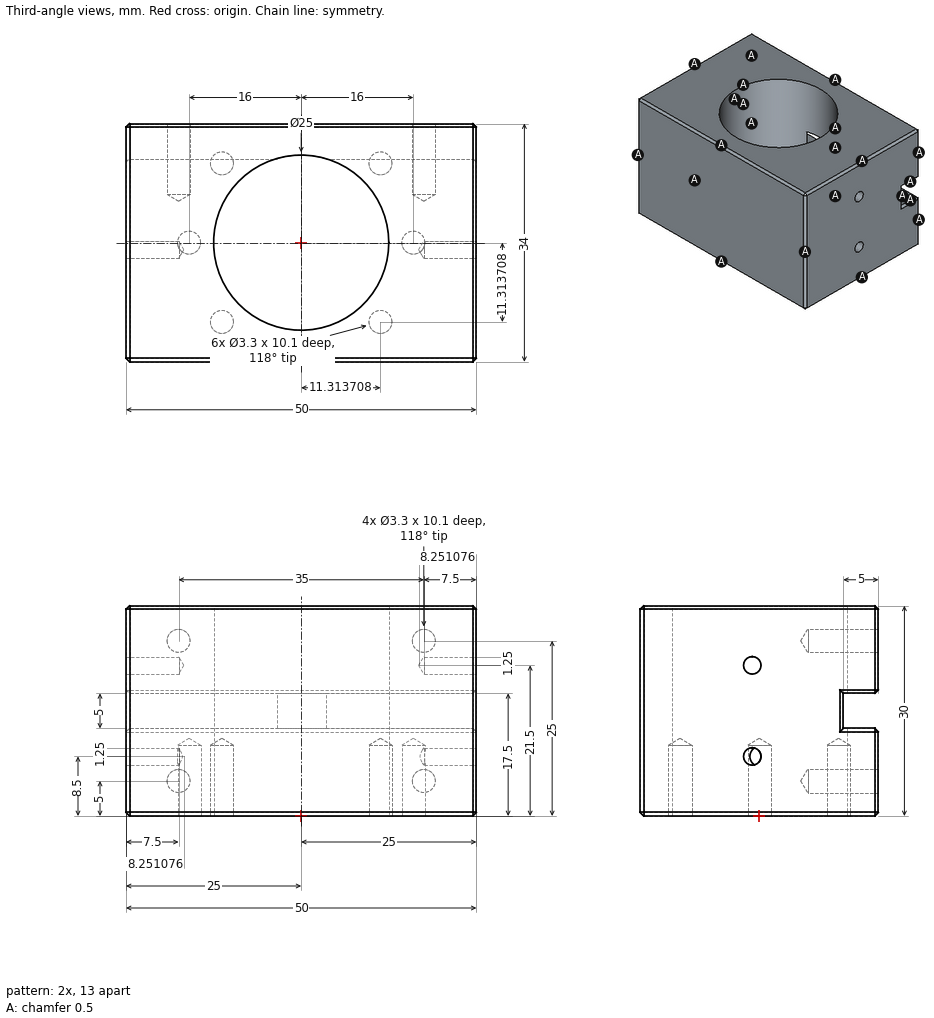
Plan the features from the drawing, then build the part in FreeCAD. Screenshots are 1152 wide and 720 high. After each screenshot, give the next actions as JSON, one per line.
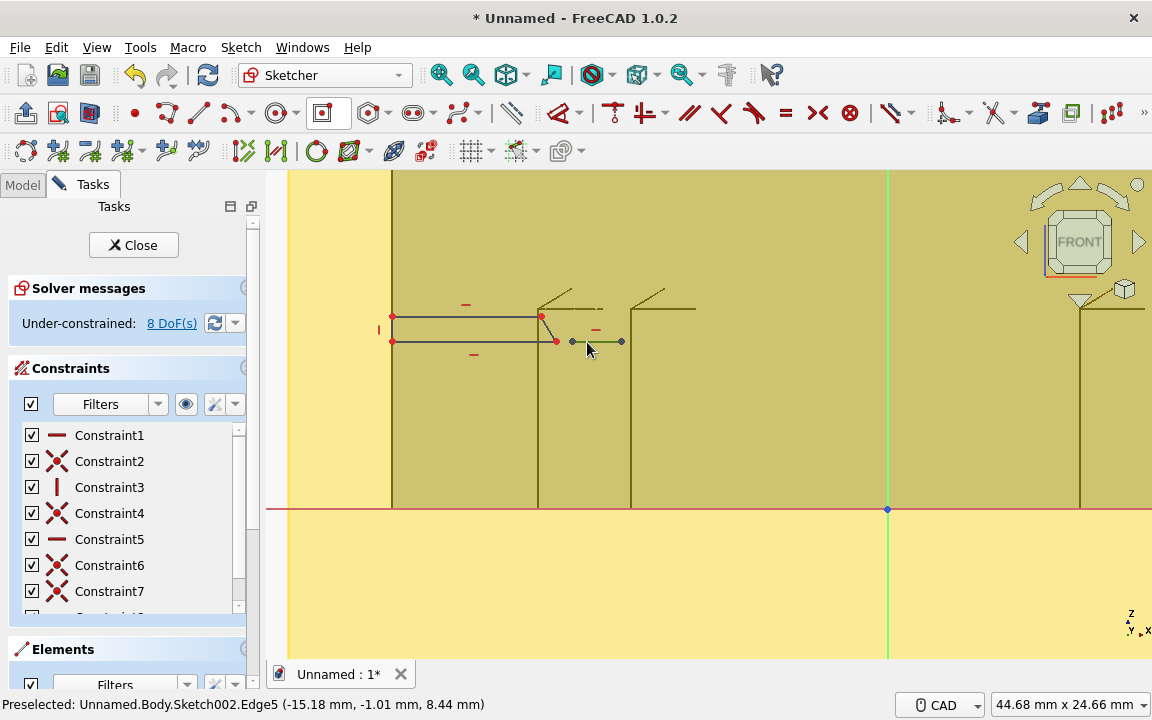
{"action": "left_click", "coordinate": [512, 114]}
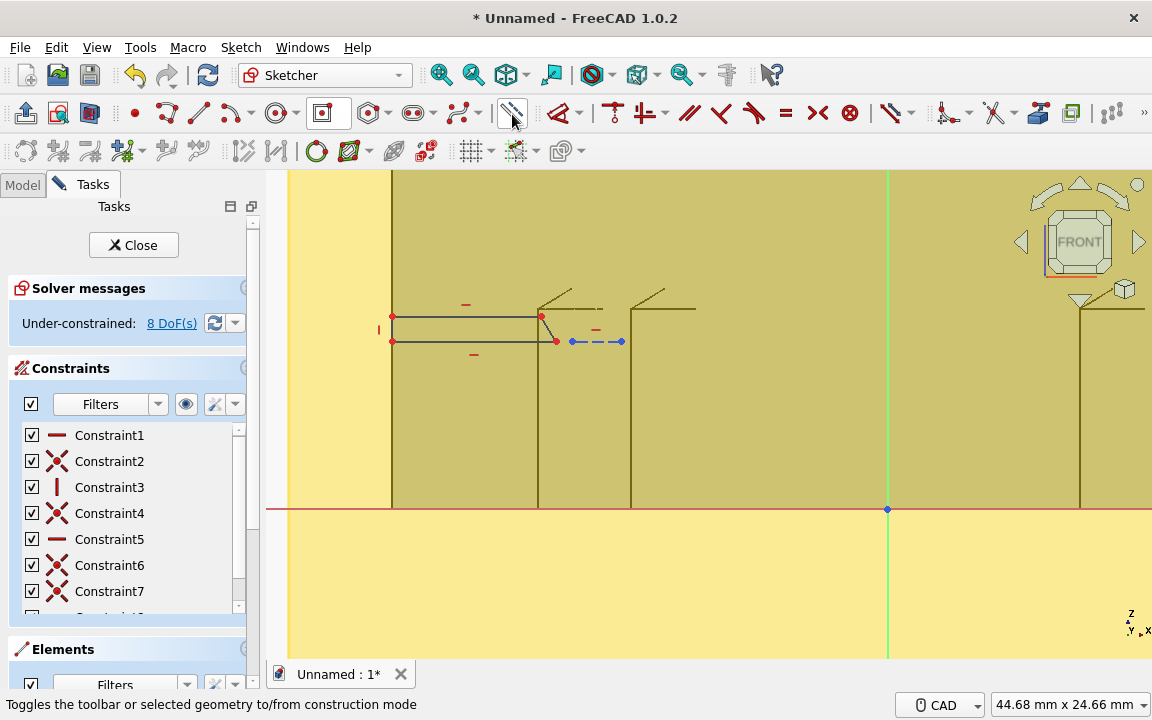
{"action": "left_click", "coordinate": [558, 114]}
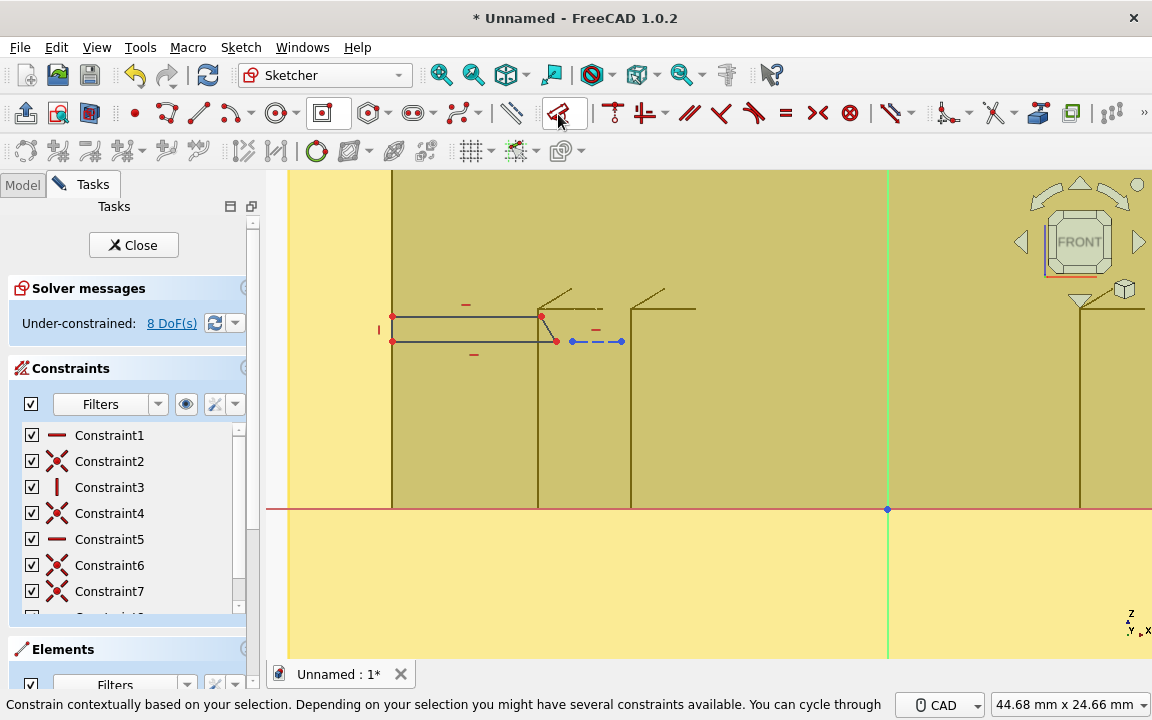
{"action": "left_click", "coordinate": [437, 317]}
{"action": "left_click", "coordinate": [466, 283]}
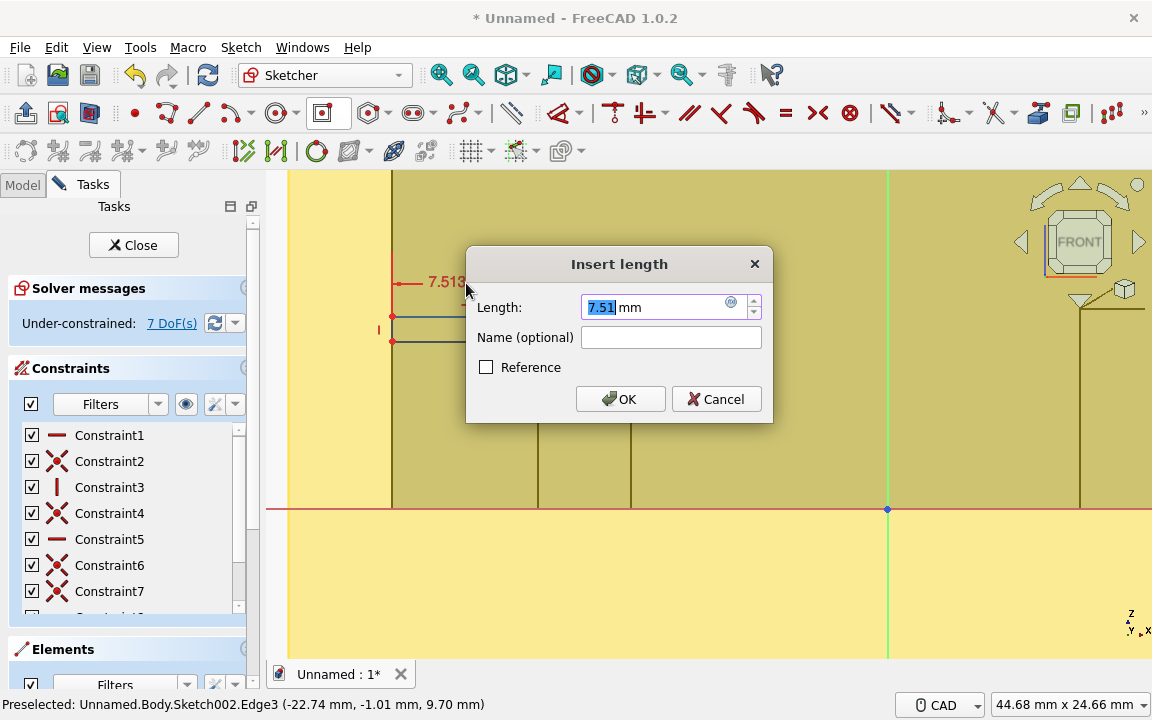
{"action": "type", "text": "7.5"}
{"action": "key", "text": "Return"}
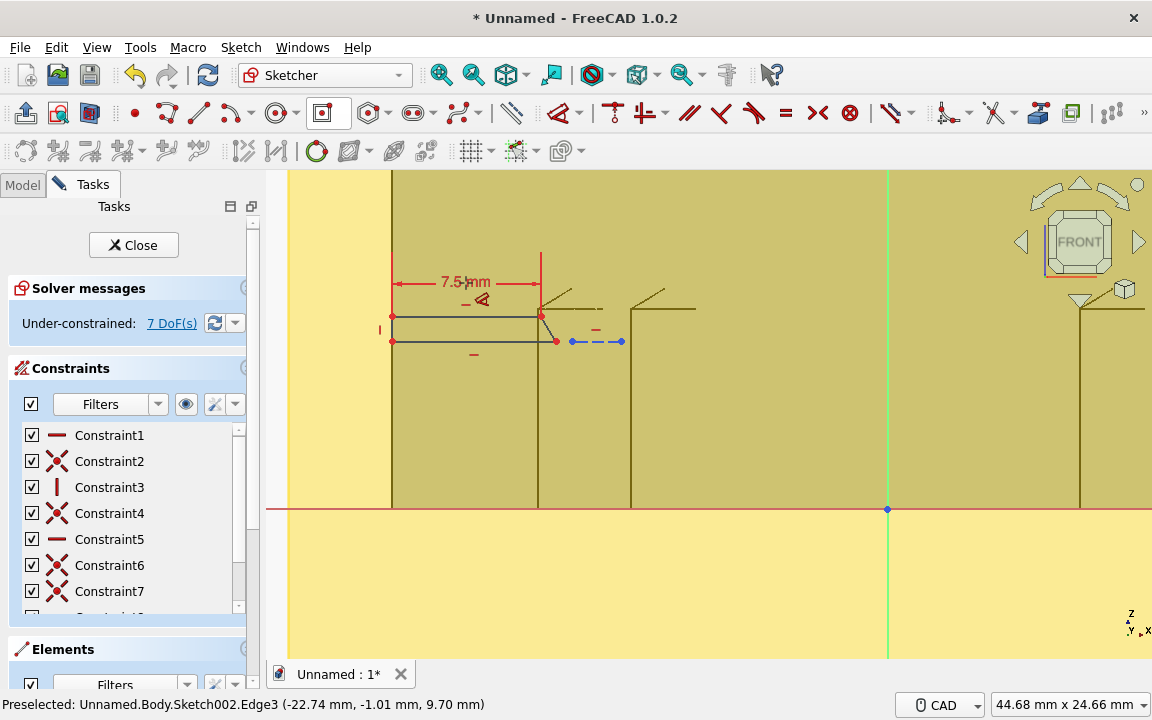
{"action": "left_click", "coordinate": [392, 342]}
{"action": "left_click", "coordinate": [640, 543]}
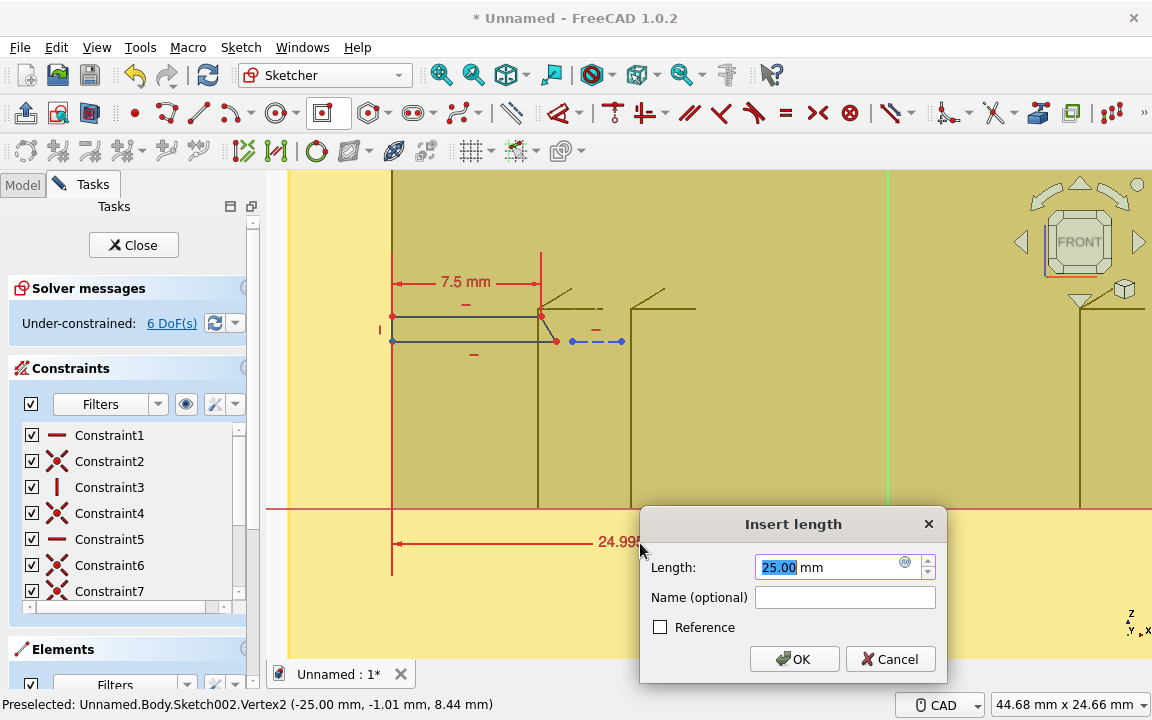
{"action": "type", "text": "25"}
{"action": "key", "text": "Return"}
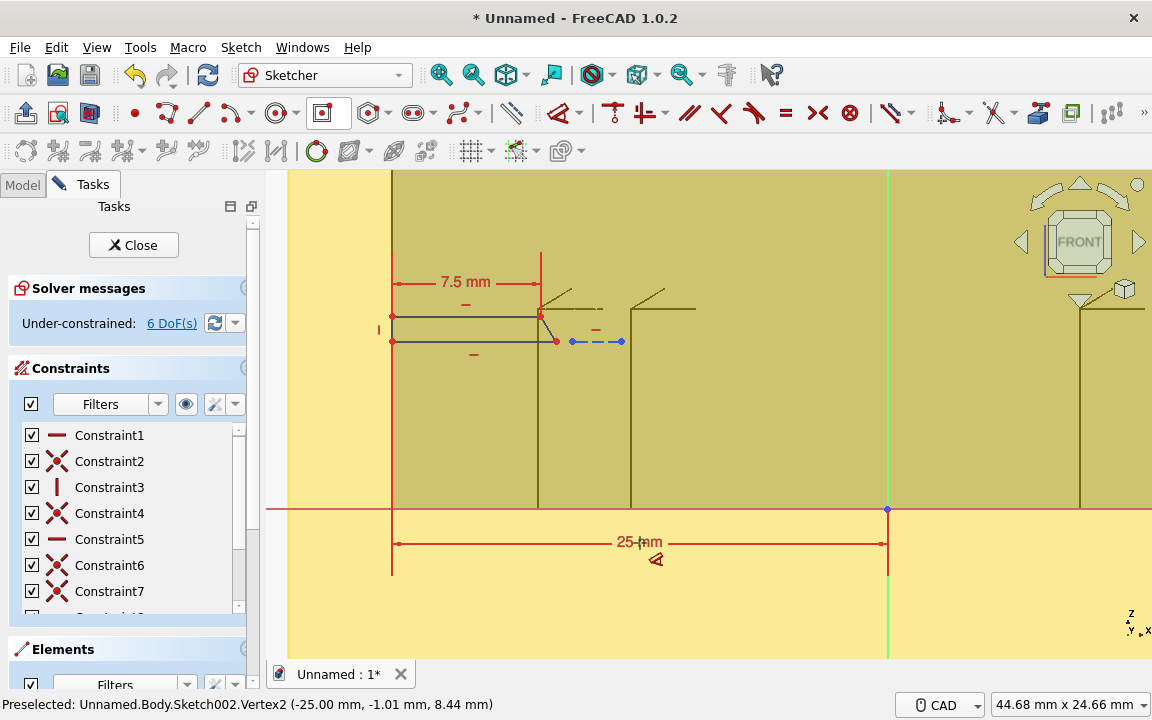
{"action": "scroll", "coordinate": [392, 332], "scroll_direction": "up", "scroll_amount": 3}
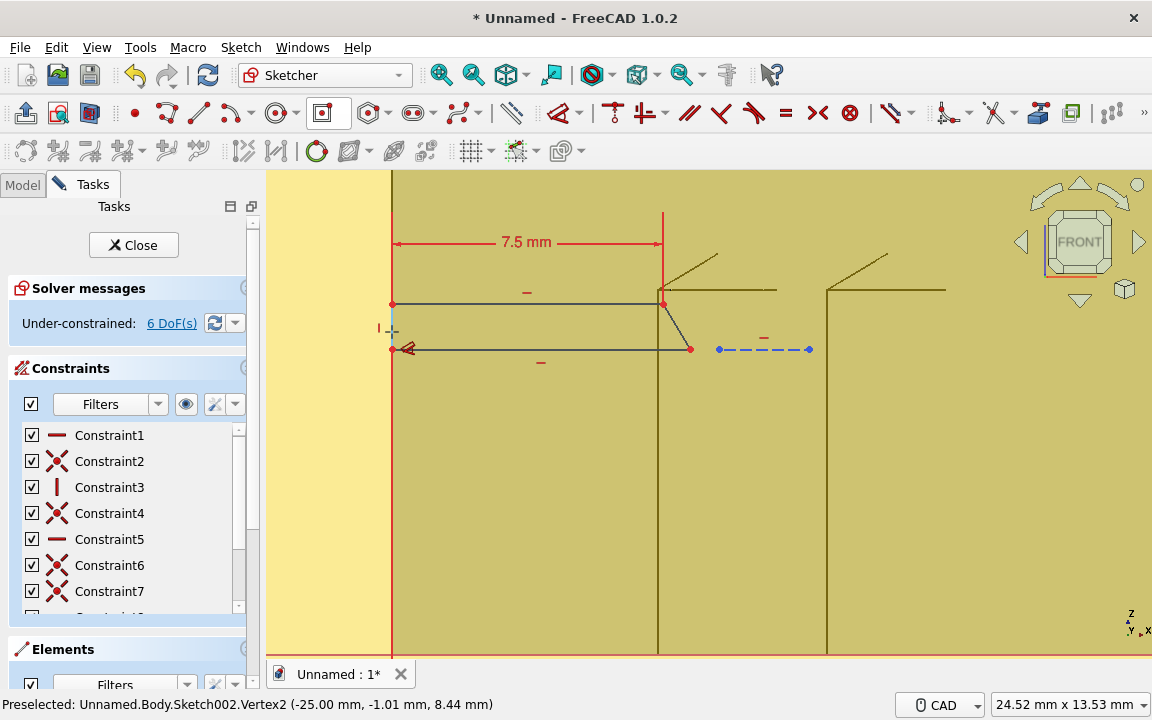
{"action": "left_click", "coordinate": [392, 332]}
{"action": "left_click", "coordinate": [358, 327]}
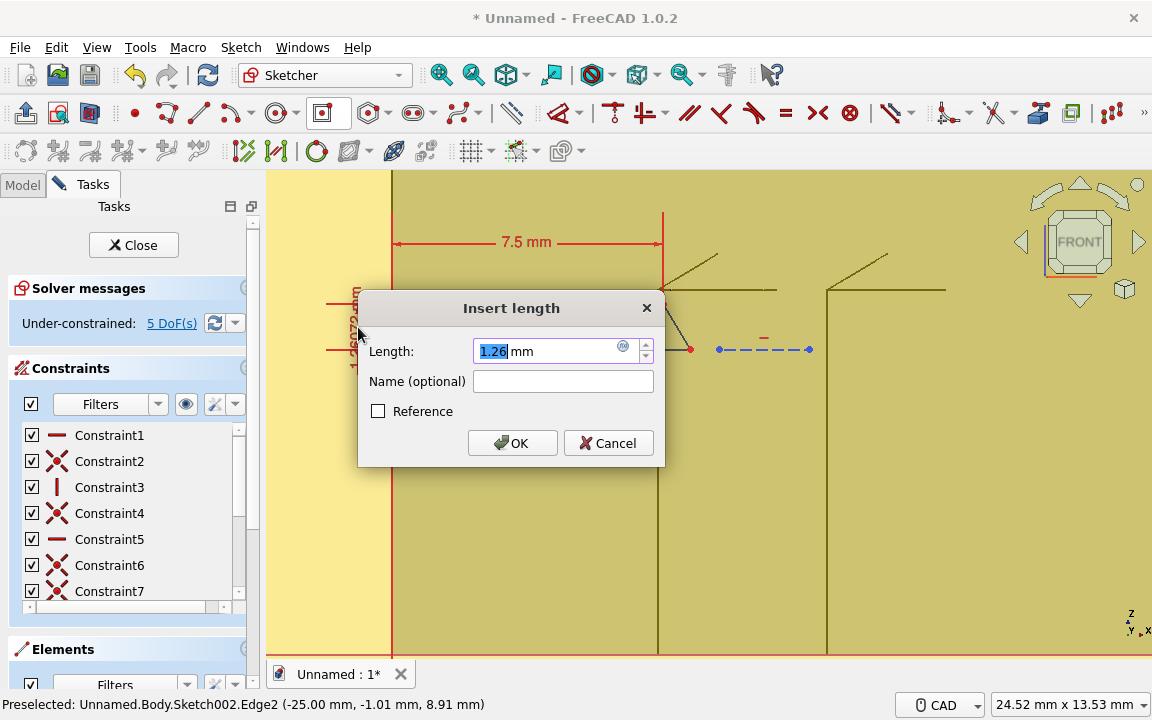
{"action": "type", "text": "1.25"}
{"action": "key", "text": "Return"}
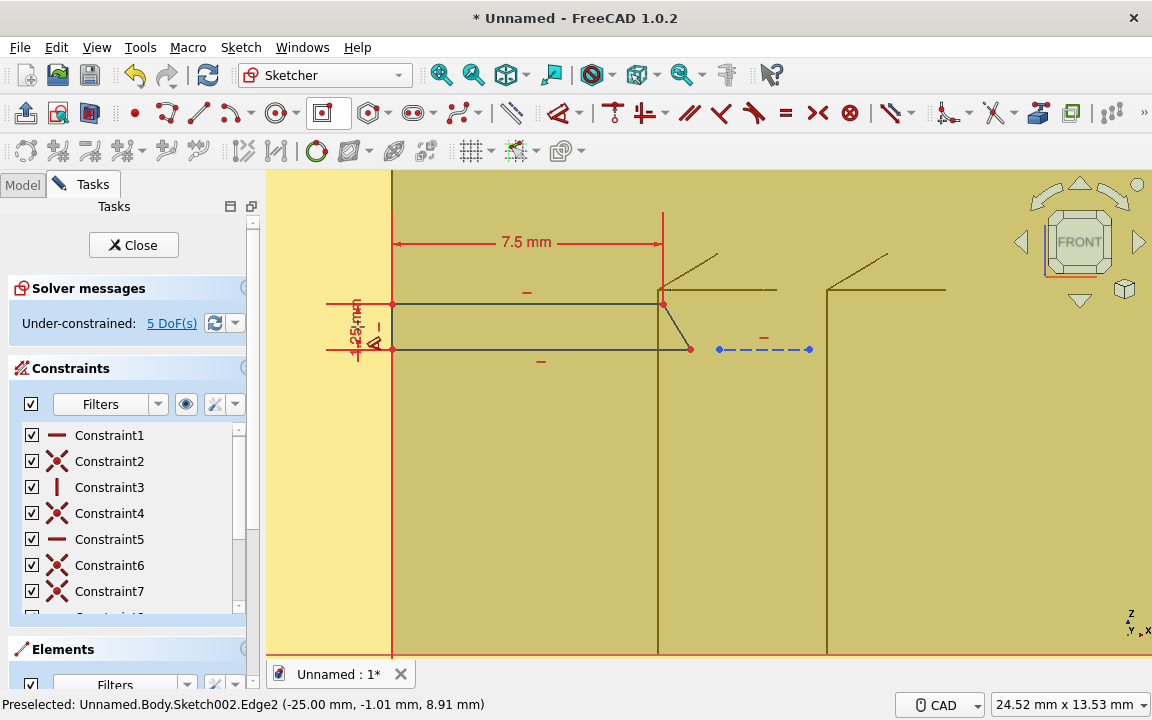
{"action": "left_click", "coordinate": [691, 350]}
{"action": "left_click", "coordinate": [657, 490]}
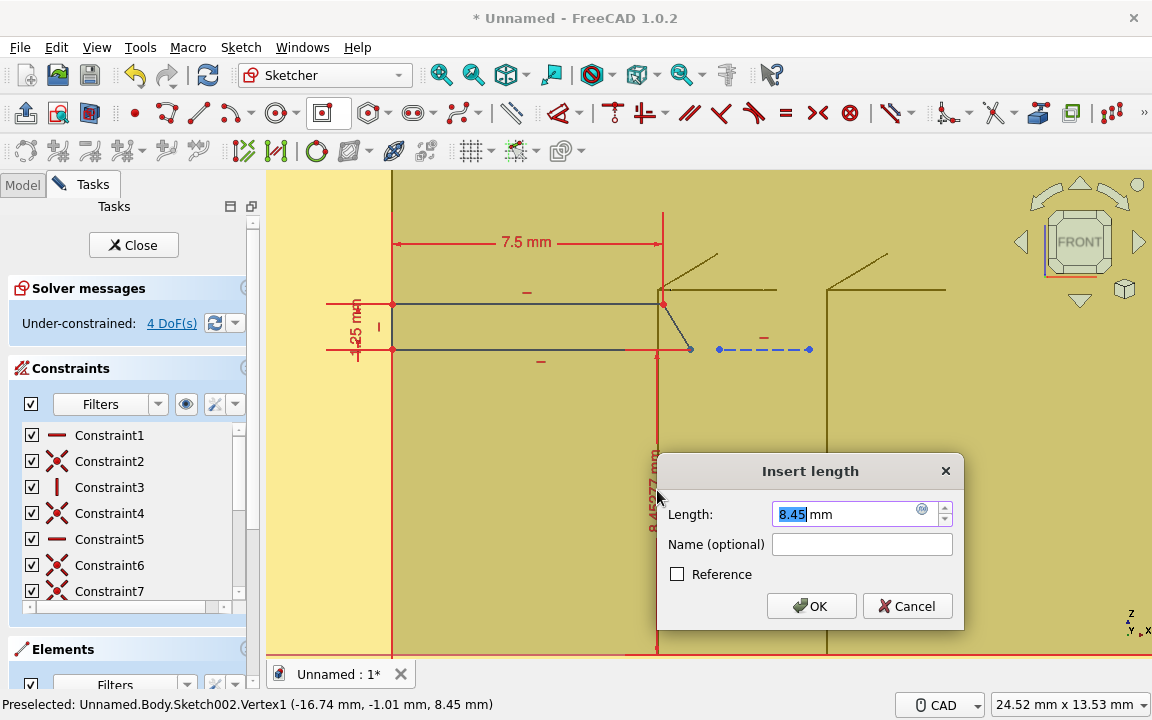
{"action": "type", "text": "8.5"}
{"action": "key", "text": "Return"}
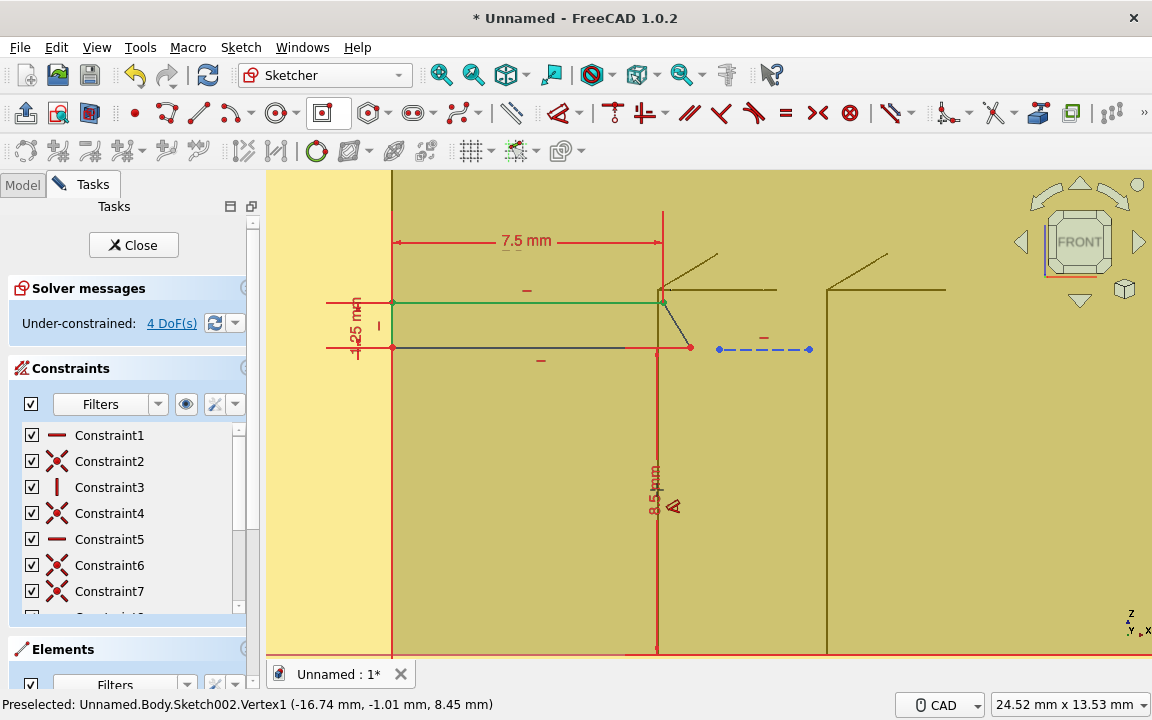
{"action": "left_click", "coordinate": [720, 350]}
{"action": "left_click", "coordinate": [686, 426]}